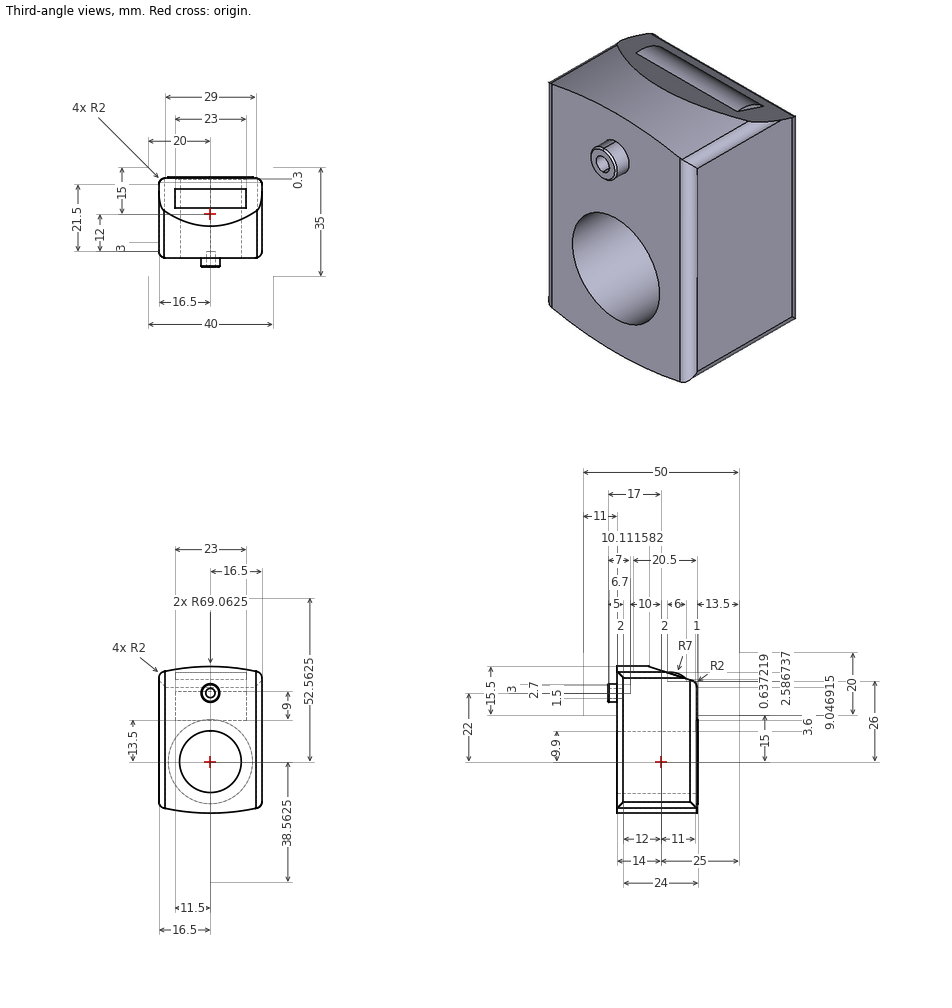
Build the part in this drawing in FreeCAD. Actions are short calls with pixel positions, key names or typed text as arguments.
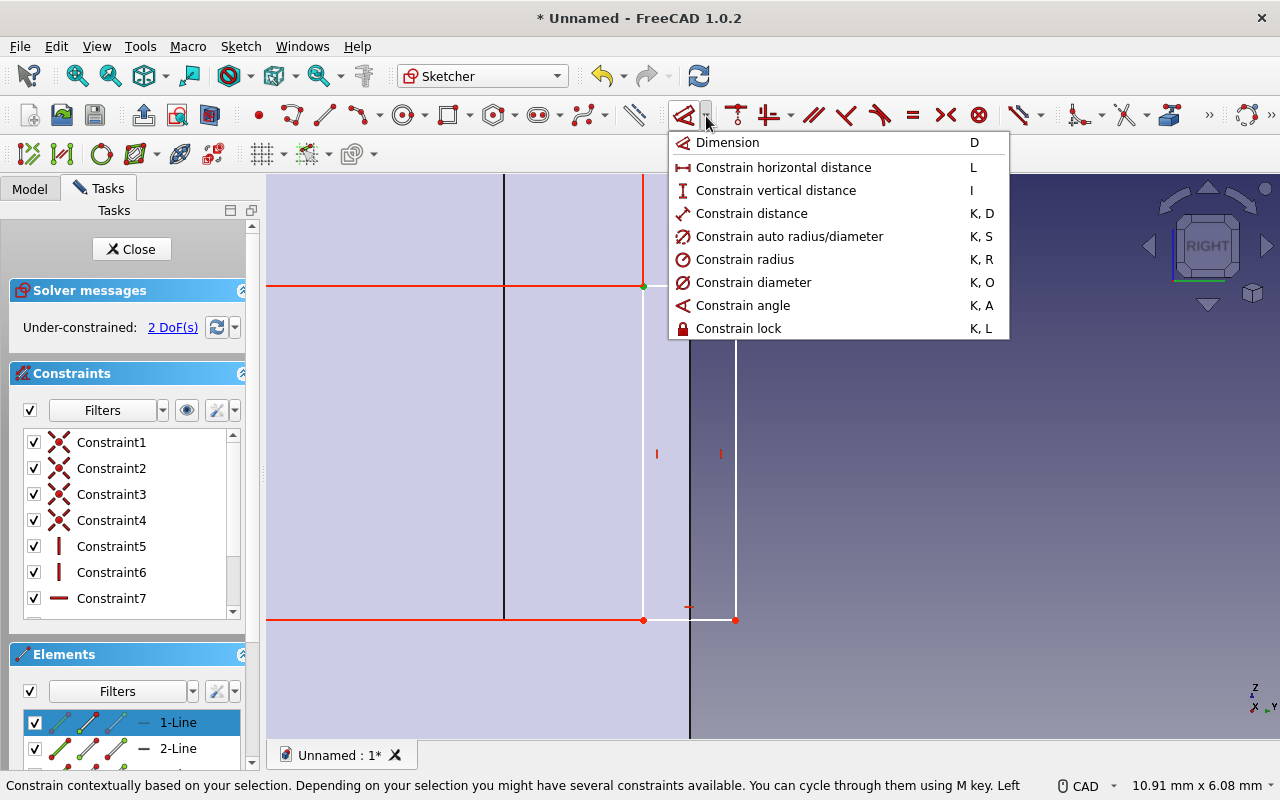
click(839, 168)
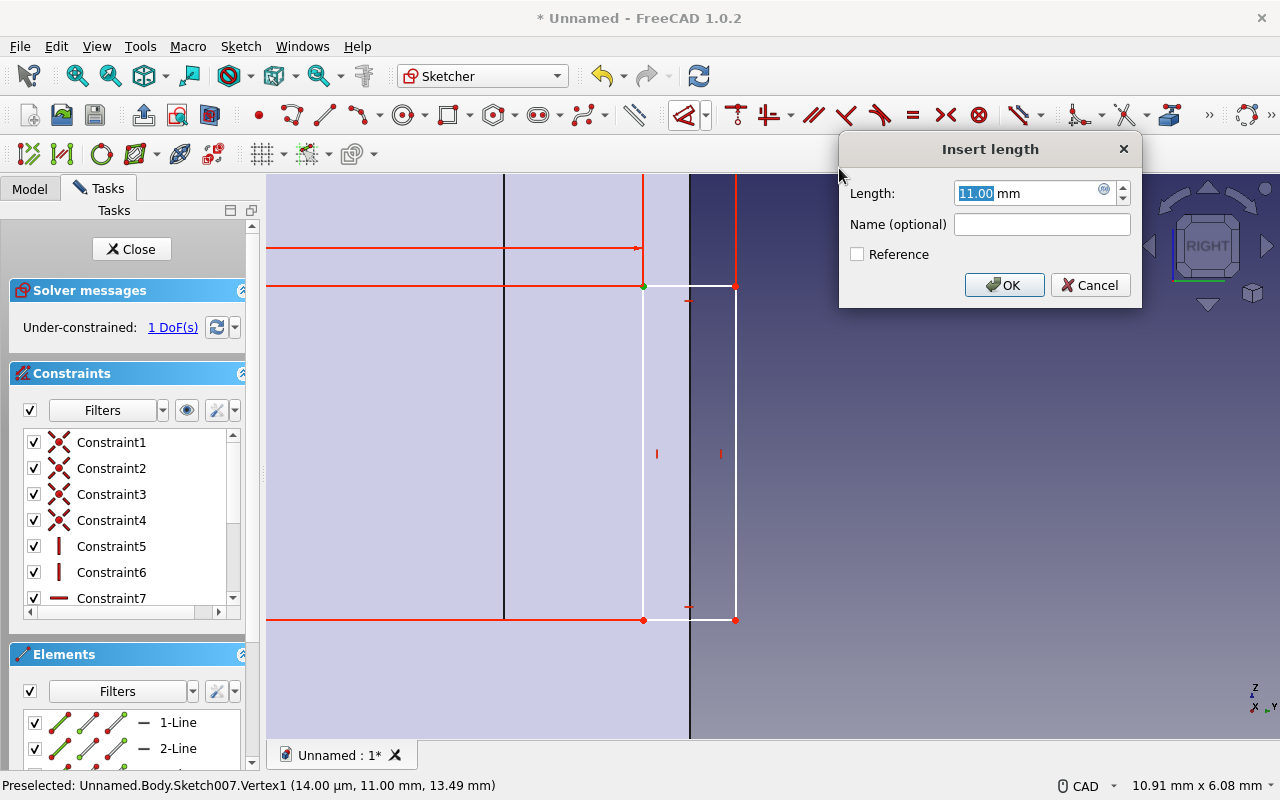
text(11)
key(Return)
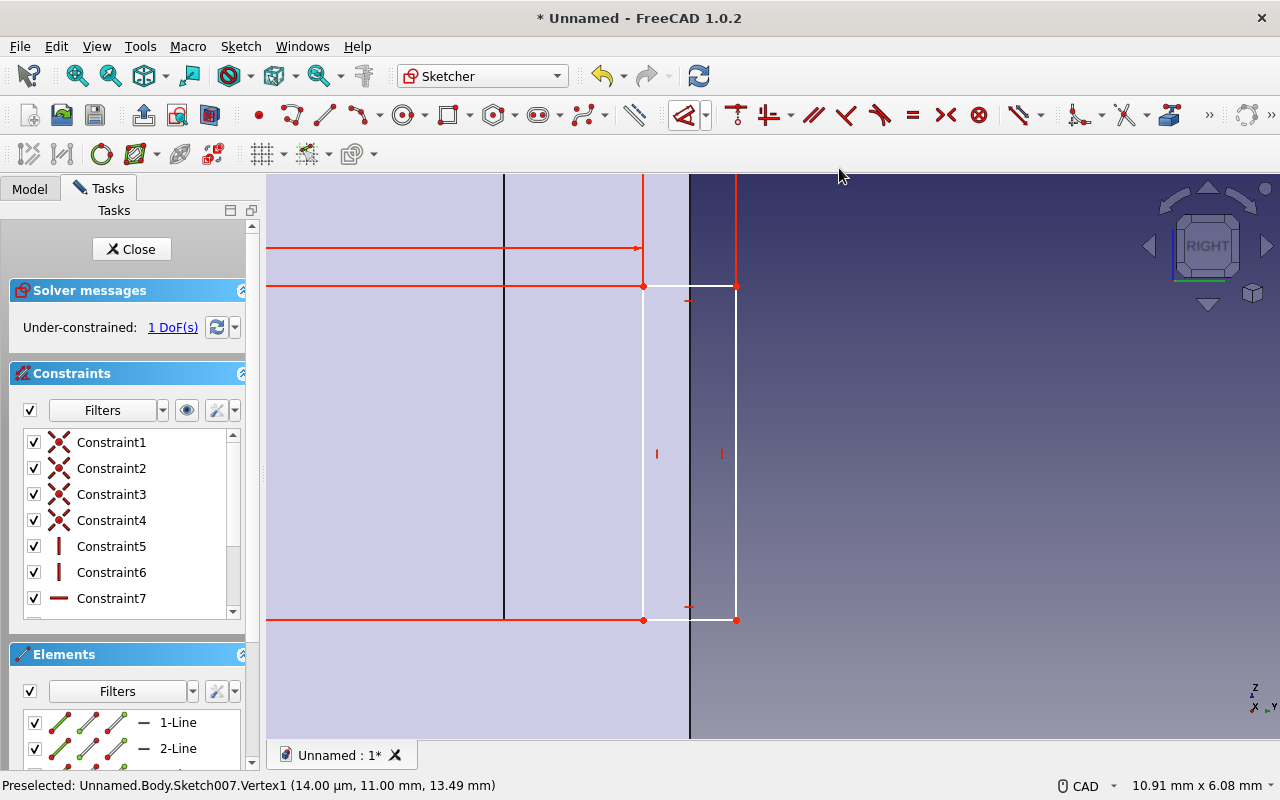
click(643, 620)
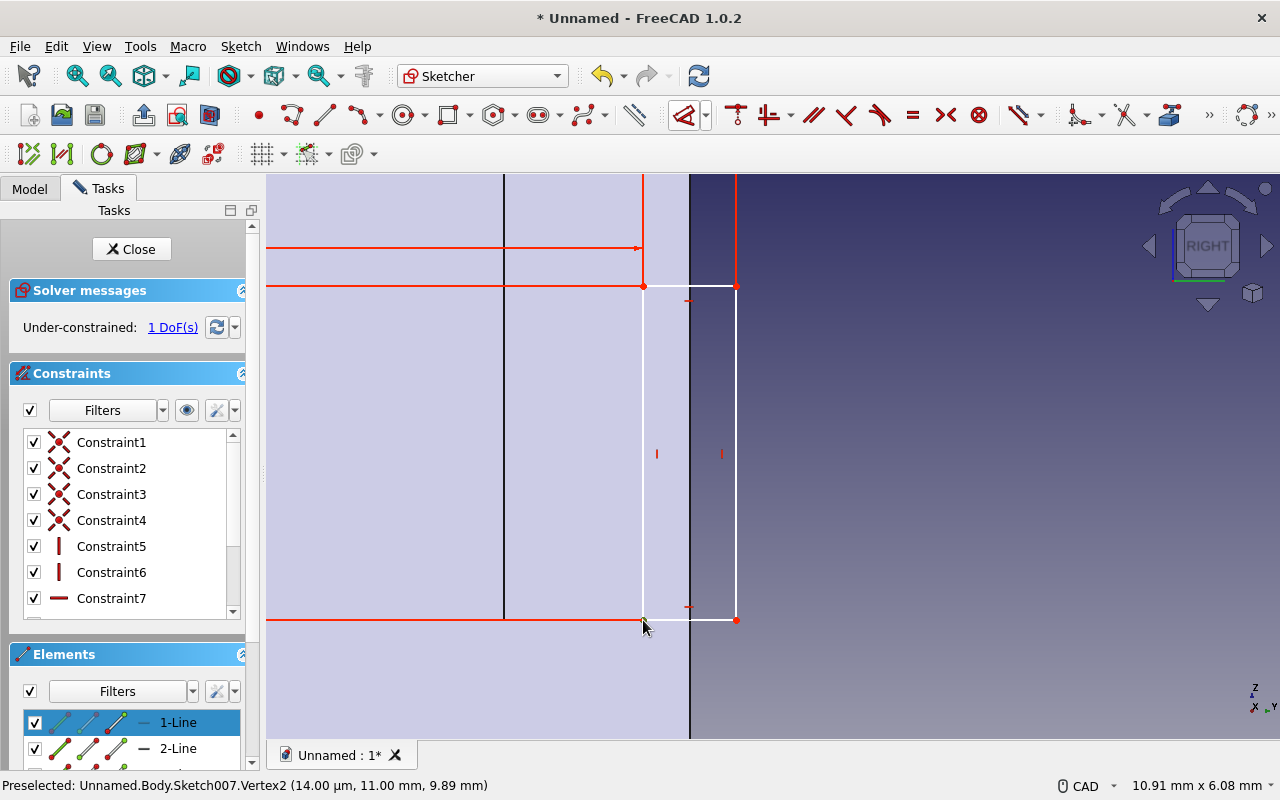
click(706, 116)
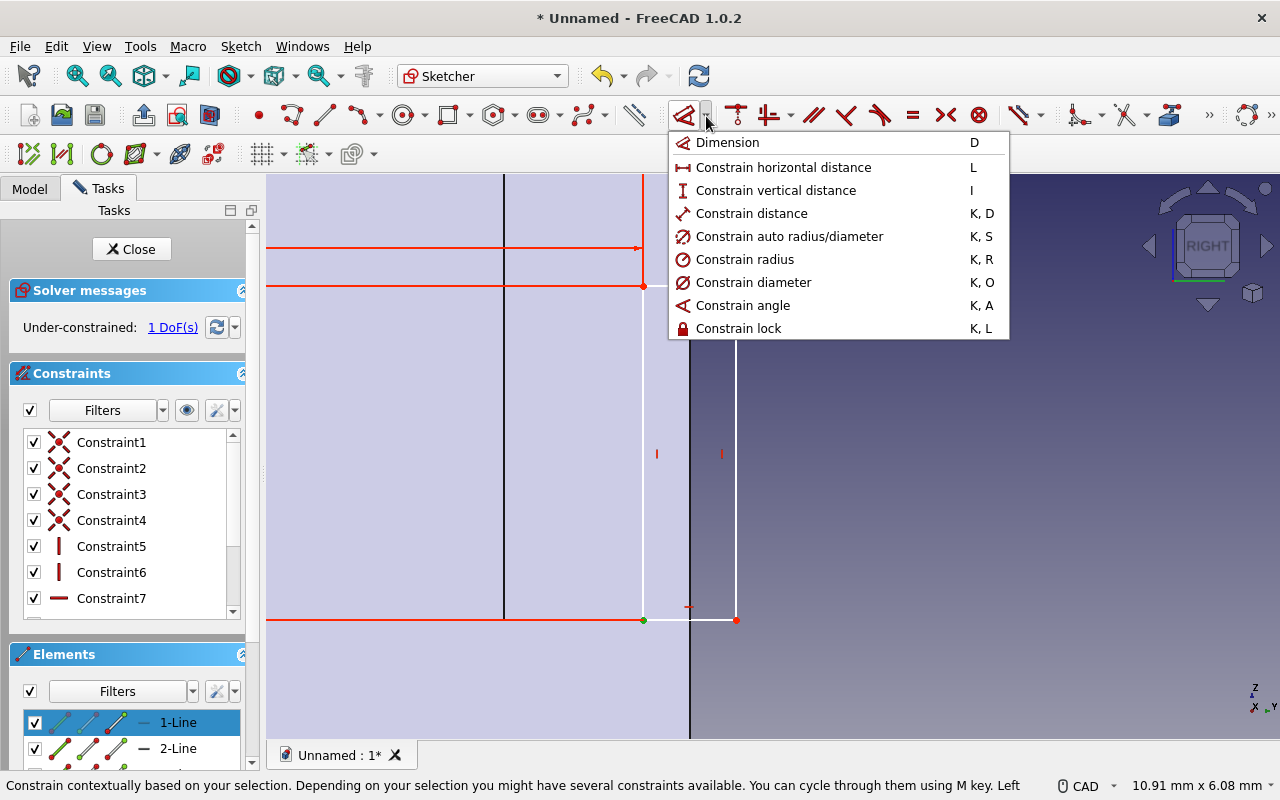
click(839, 190)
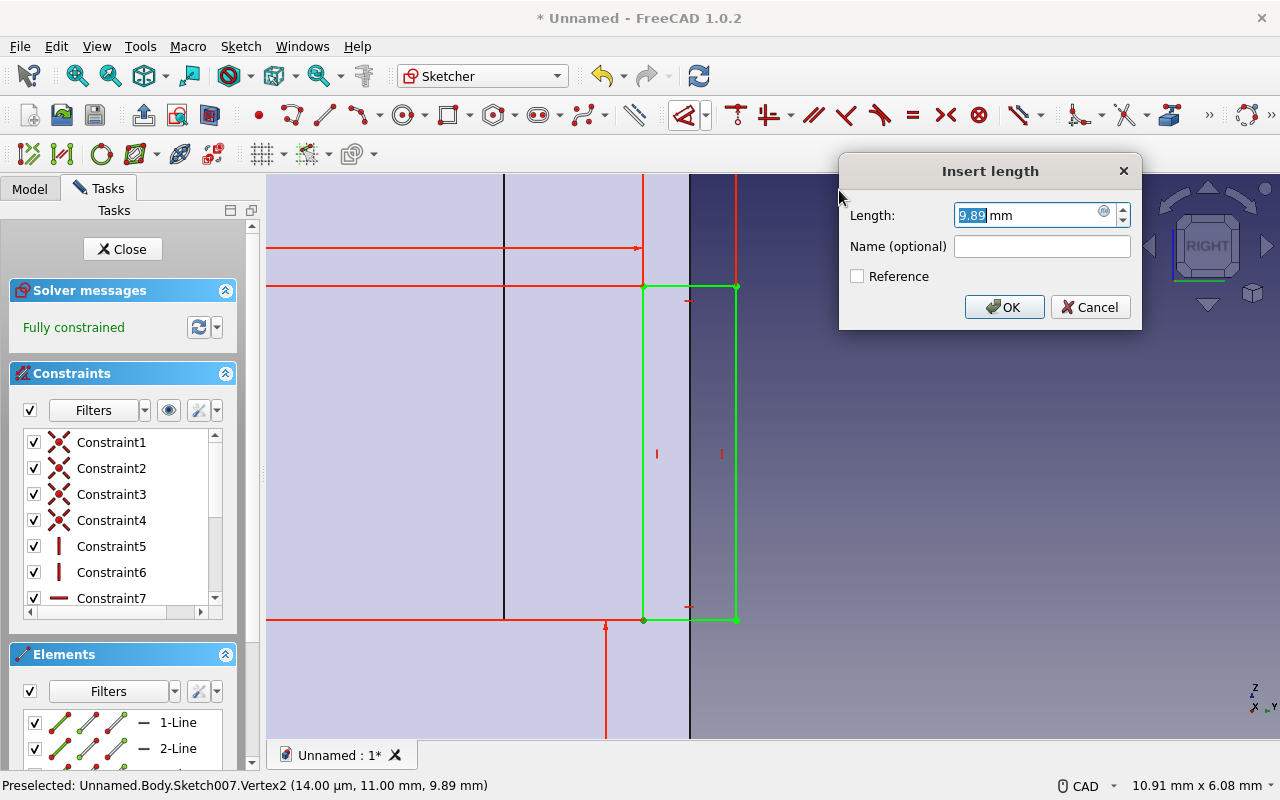
text(9.9)
key(Return)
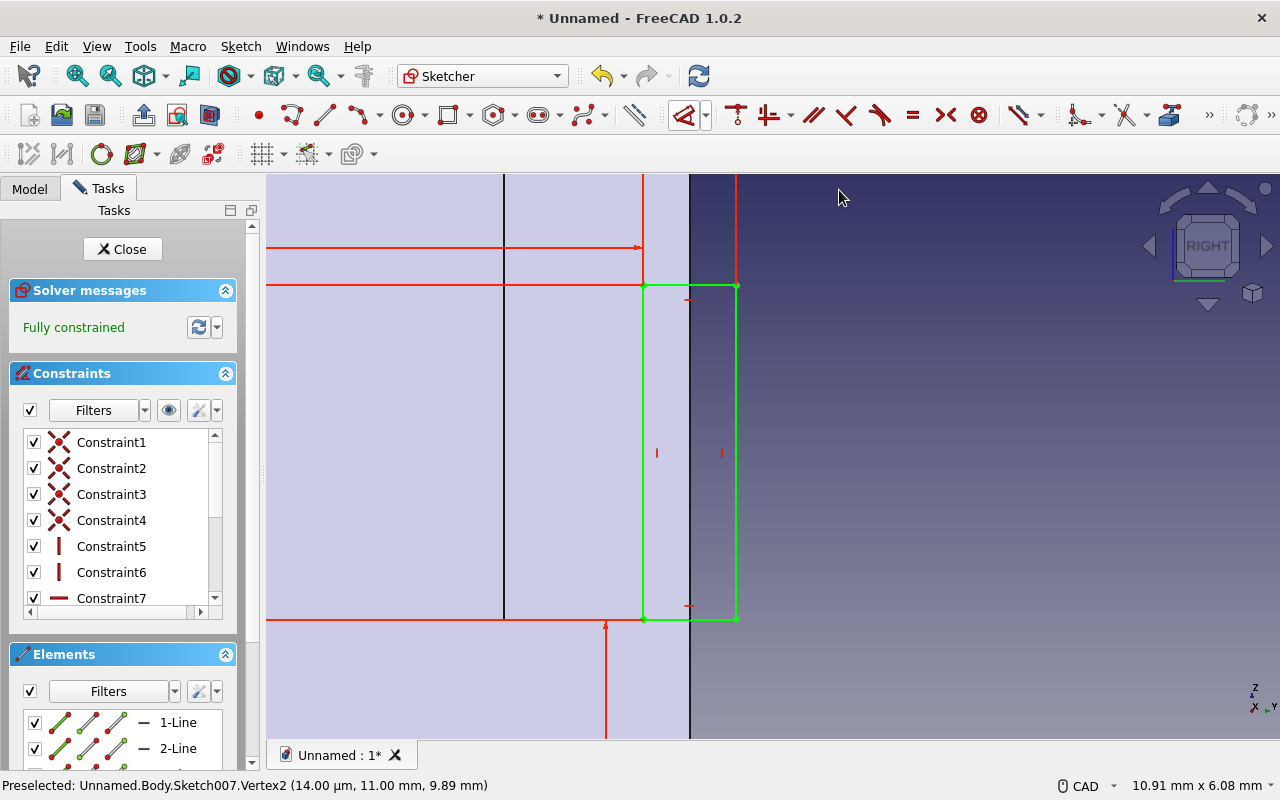
click(123, 249)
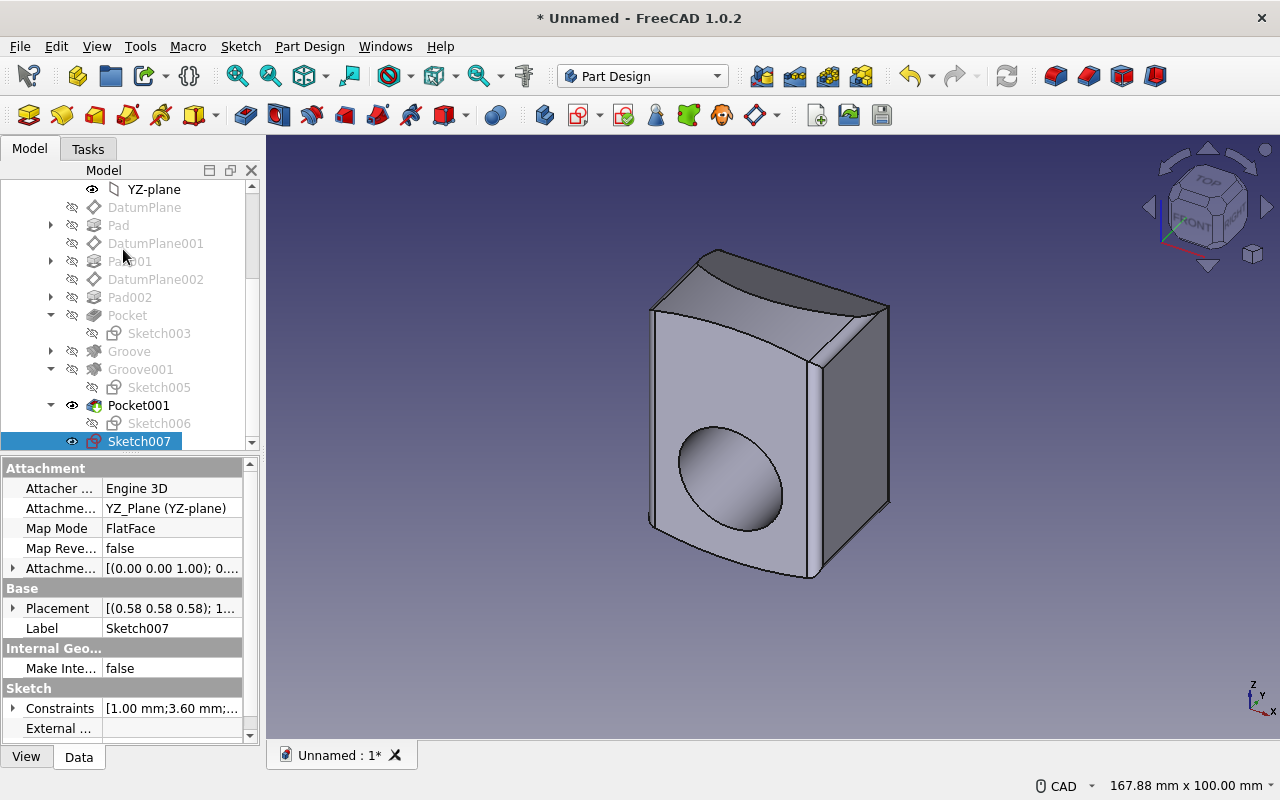
click(62, 116)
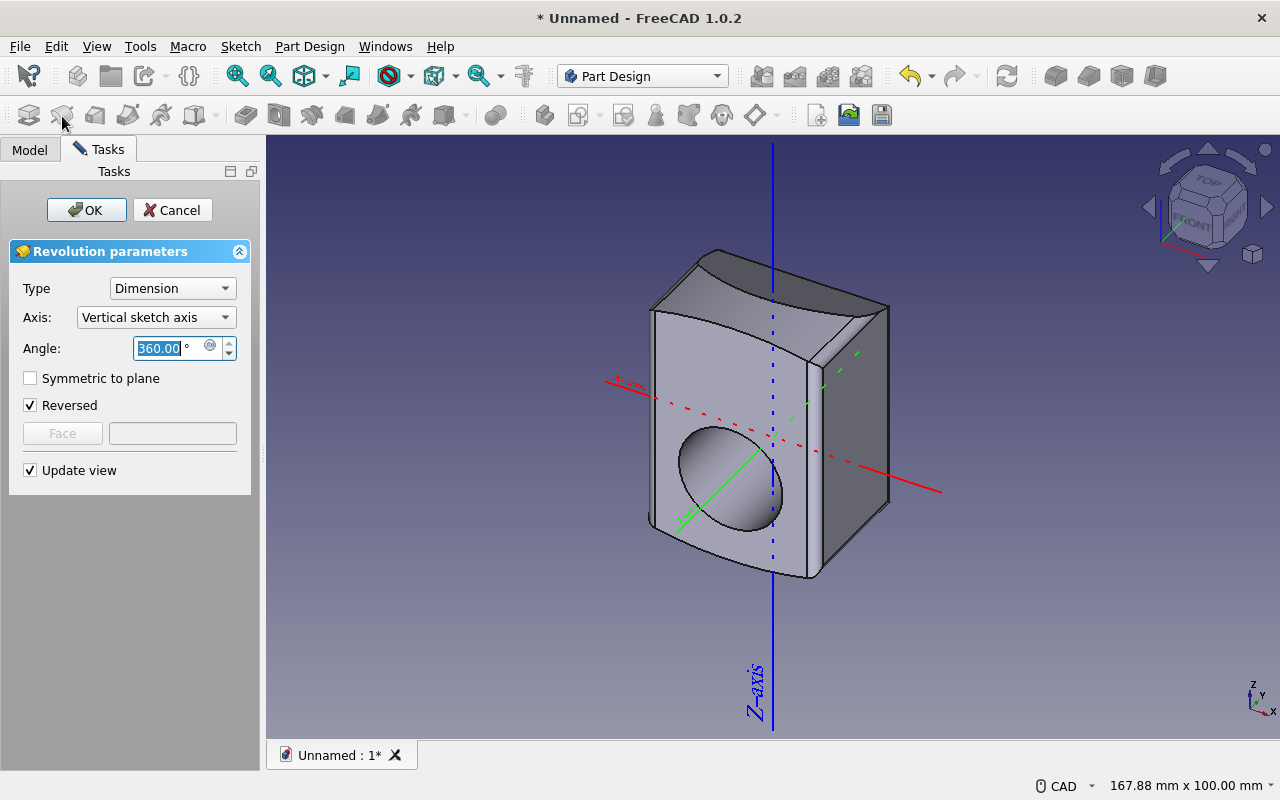
click(157, 318)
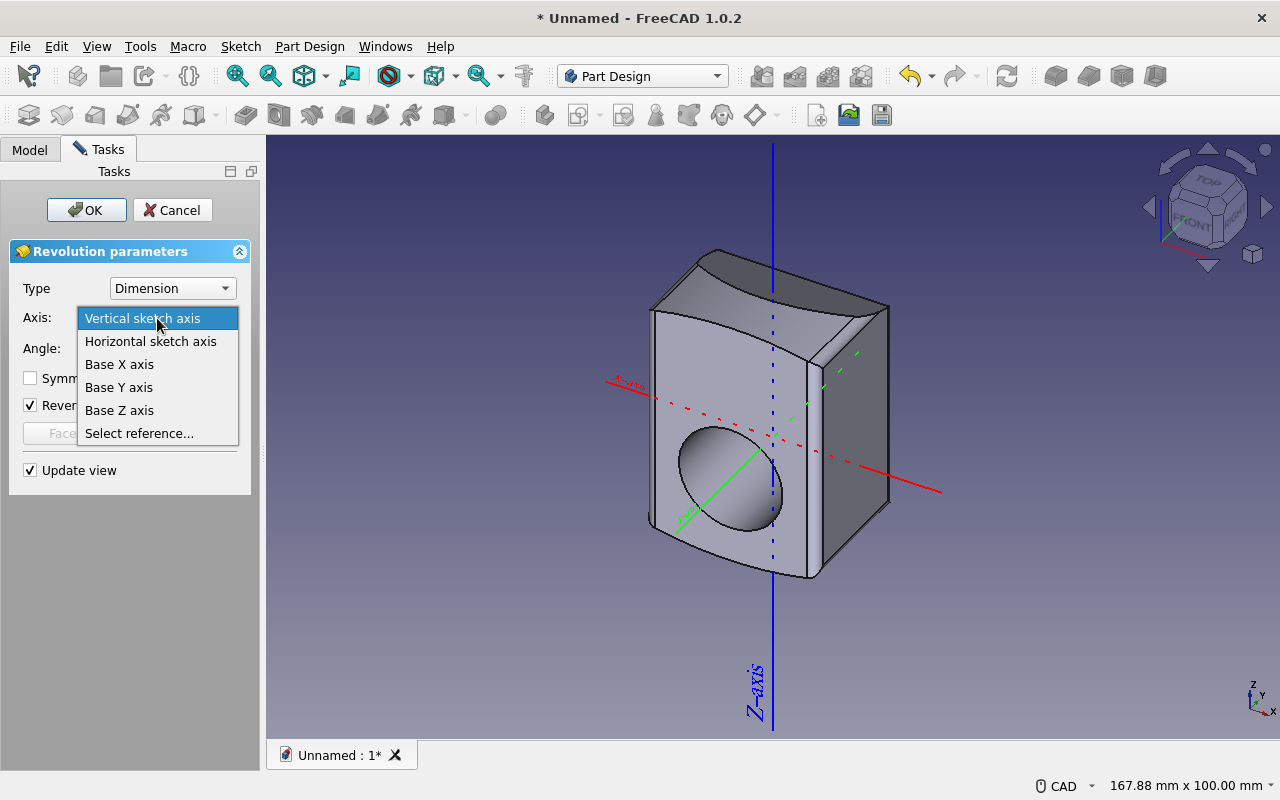
click(156, 342)